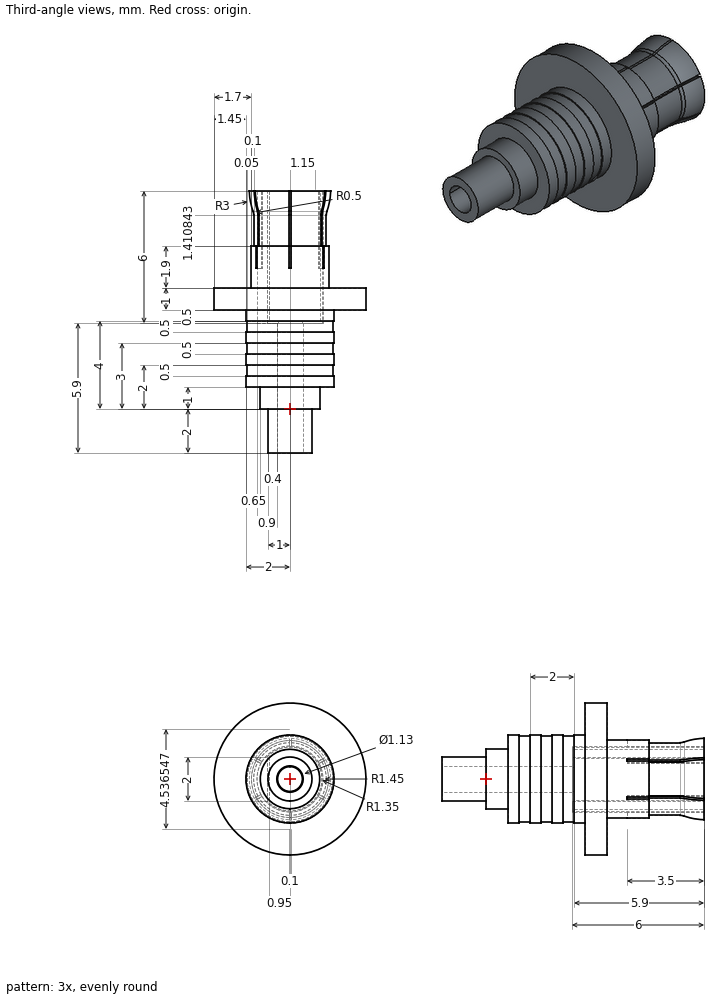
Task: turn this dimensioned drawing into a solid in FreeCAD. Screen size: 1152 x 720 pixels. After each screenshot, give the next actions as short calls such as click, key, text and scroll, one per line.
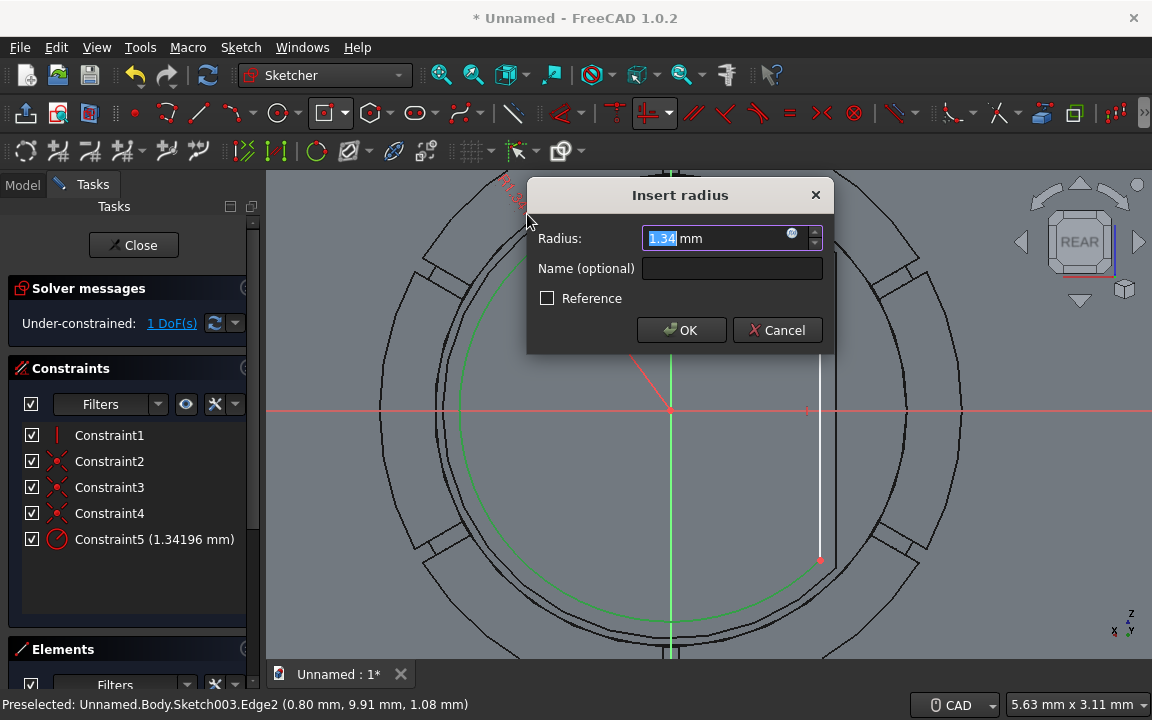
text(1.35)
key(Return)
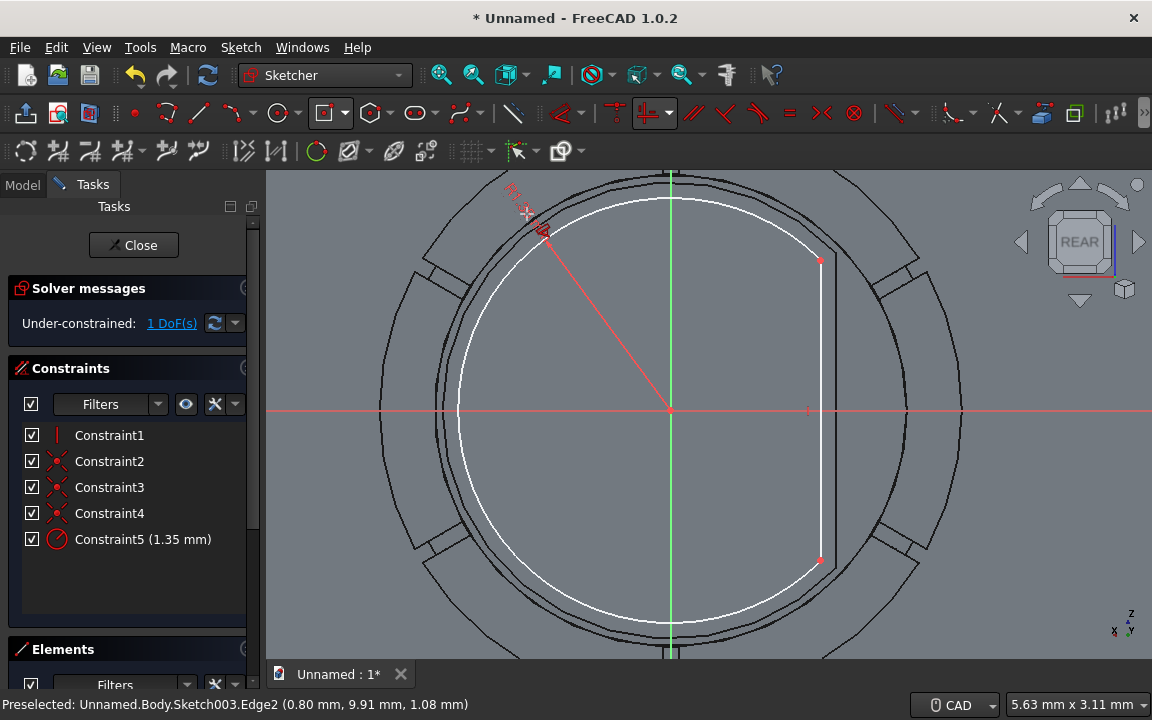
click(821, 561)
click(746, 595)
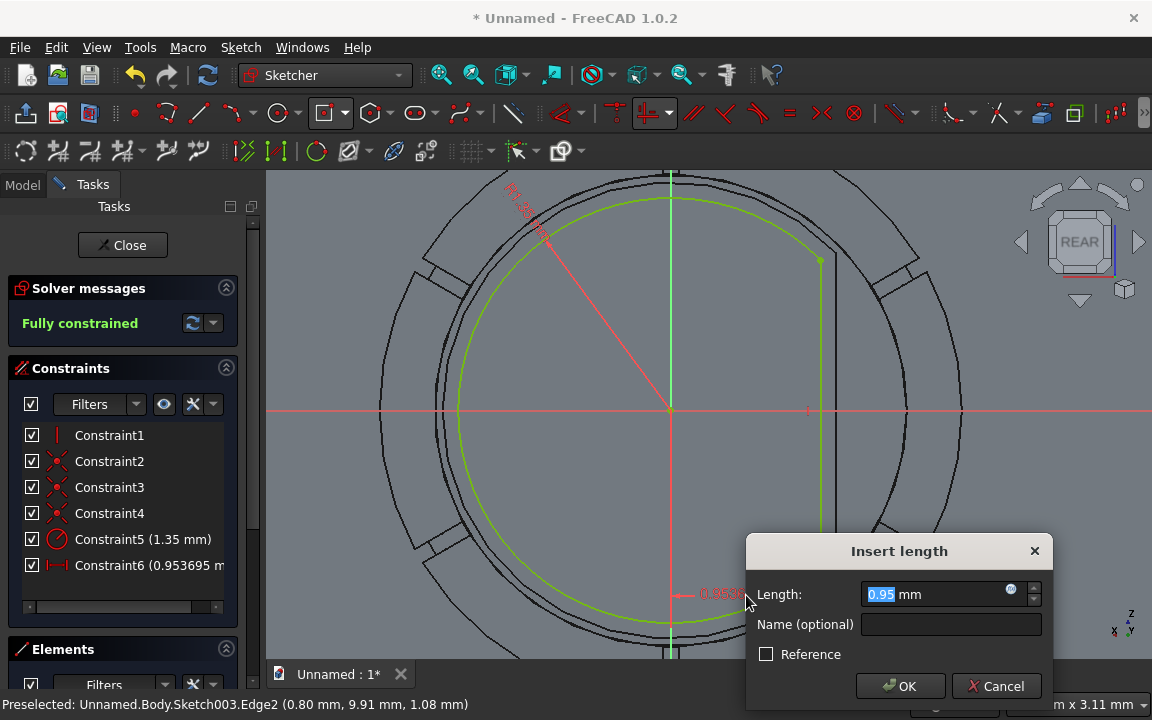
text(0.95)
key(Return)
key(Escape)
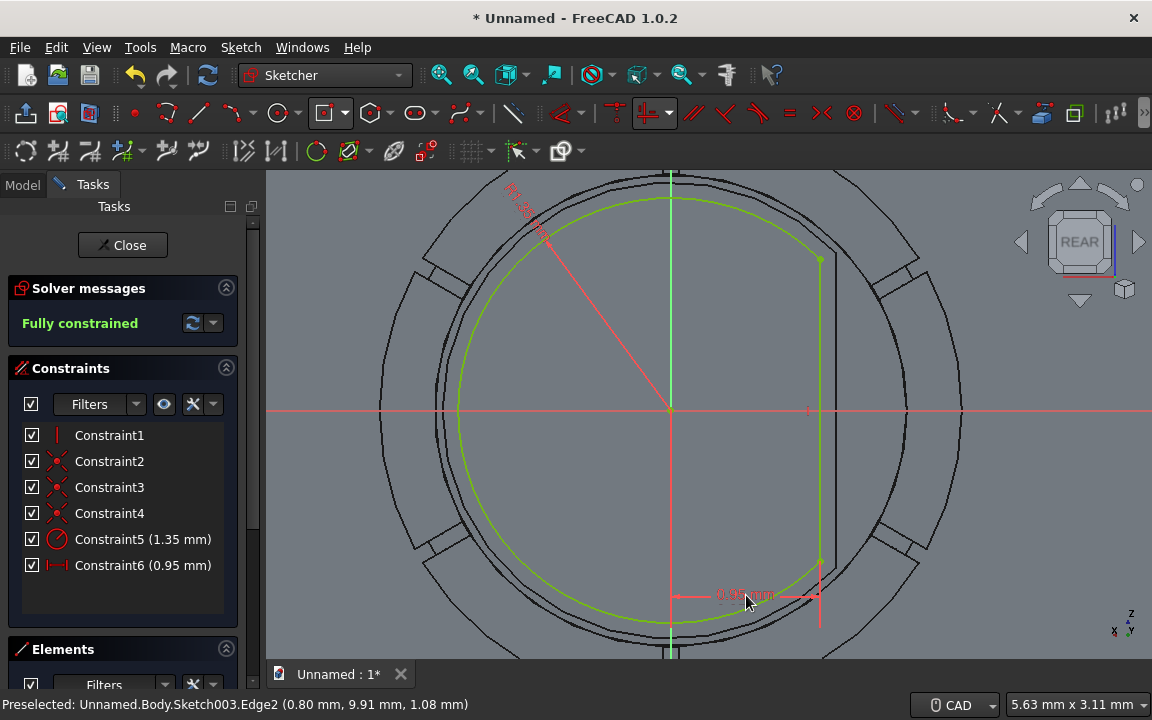
click(123, 245)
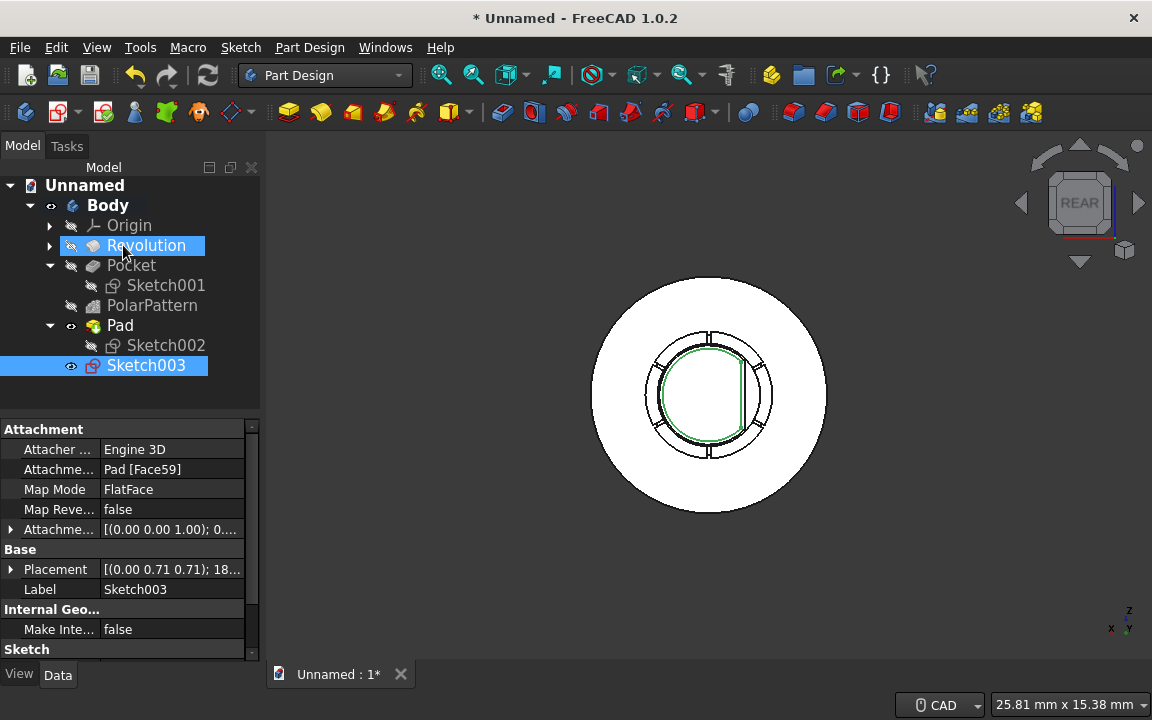
click(504, 112)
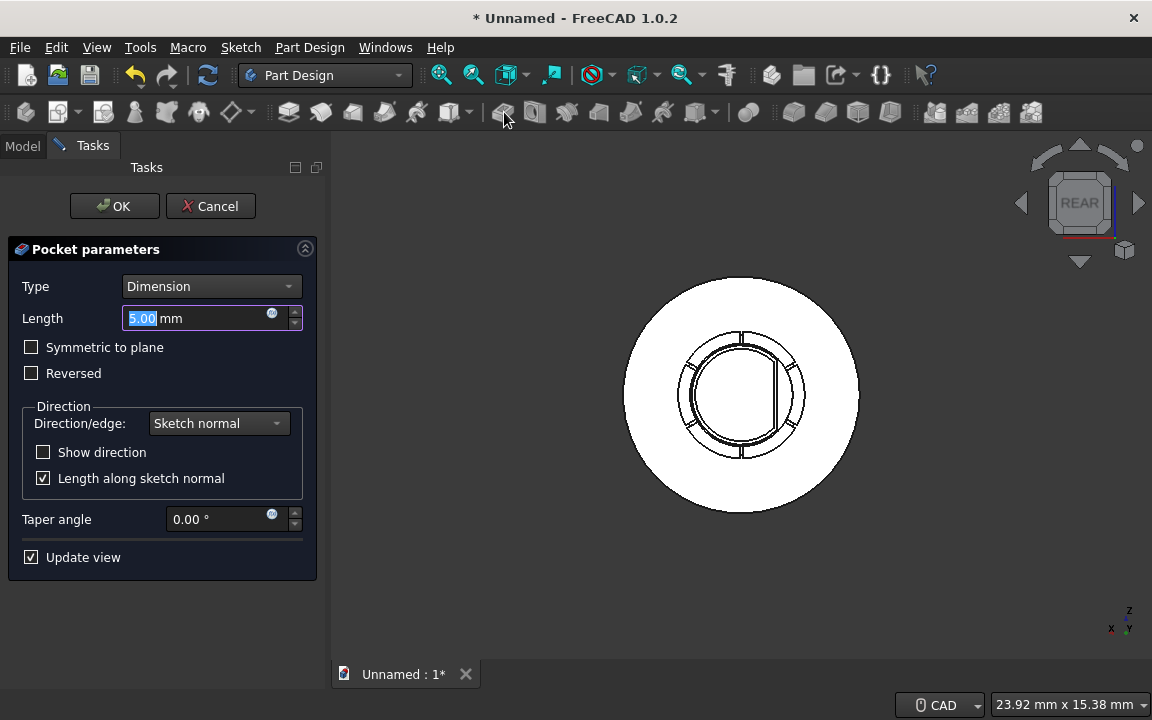
text(5.9)
key(Tab)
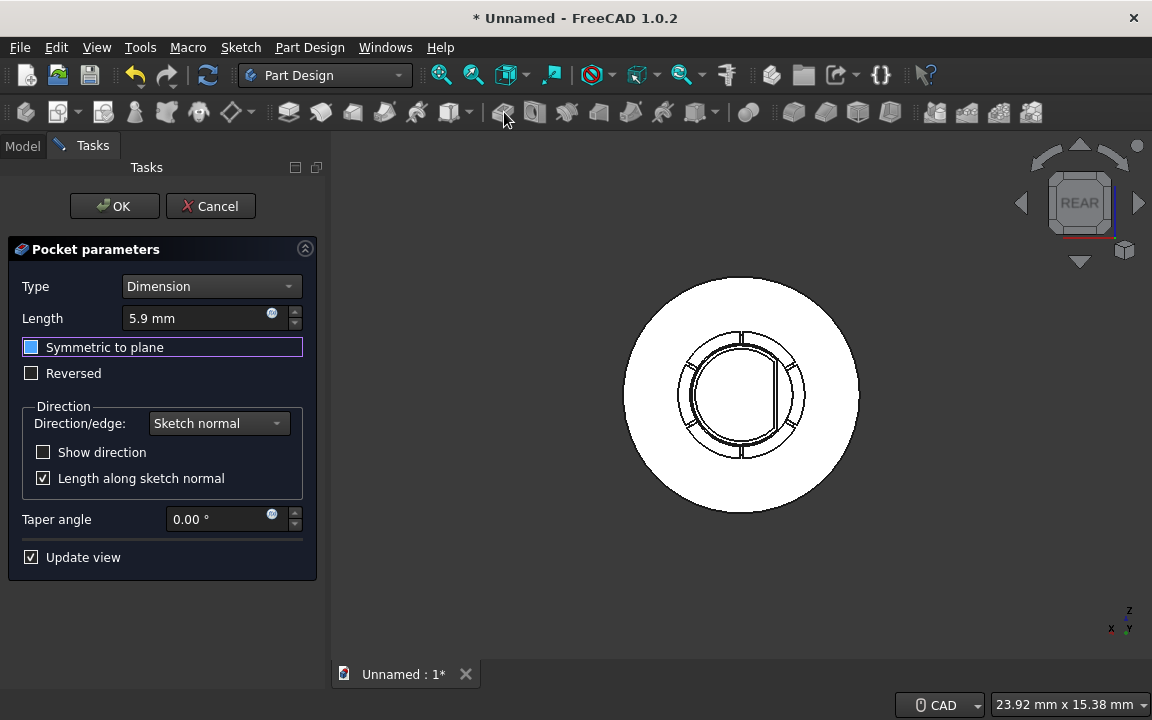
click(115, 206)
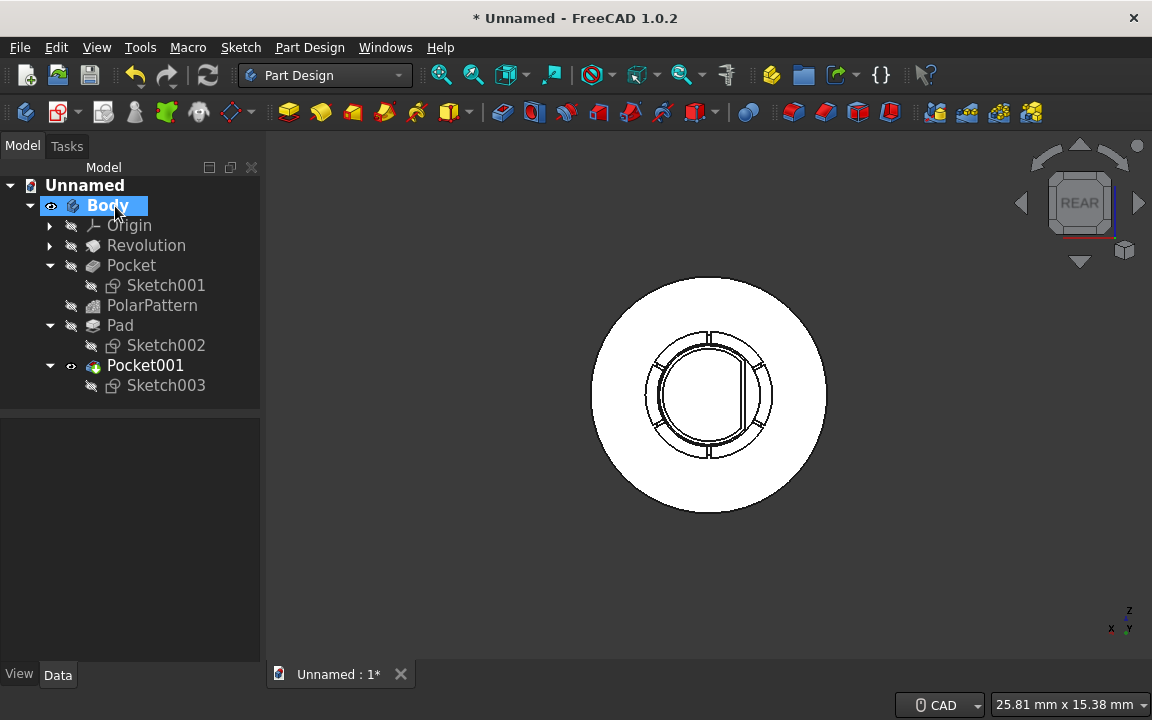
click(442, 76)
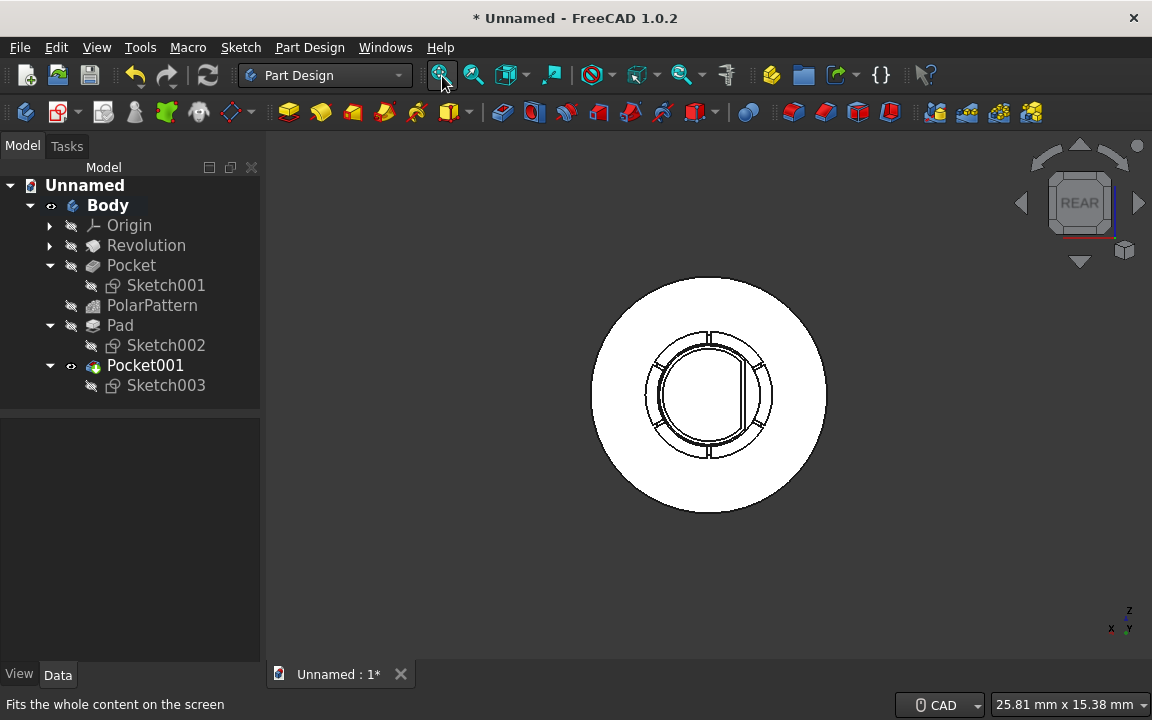
click(702, 394)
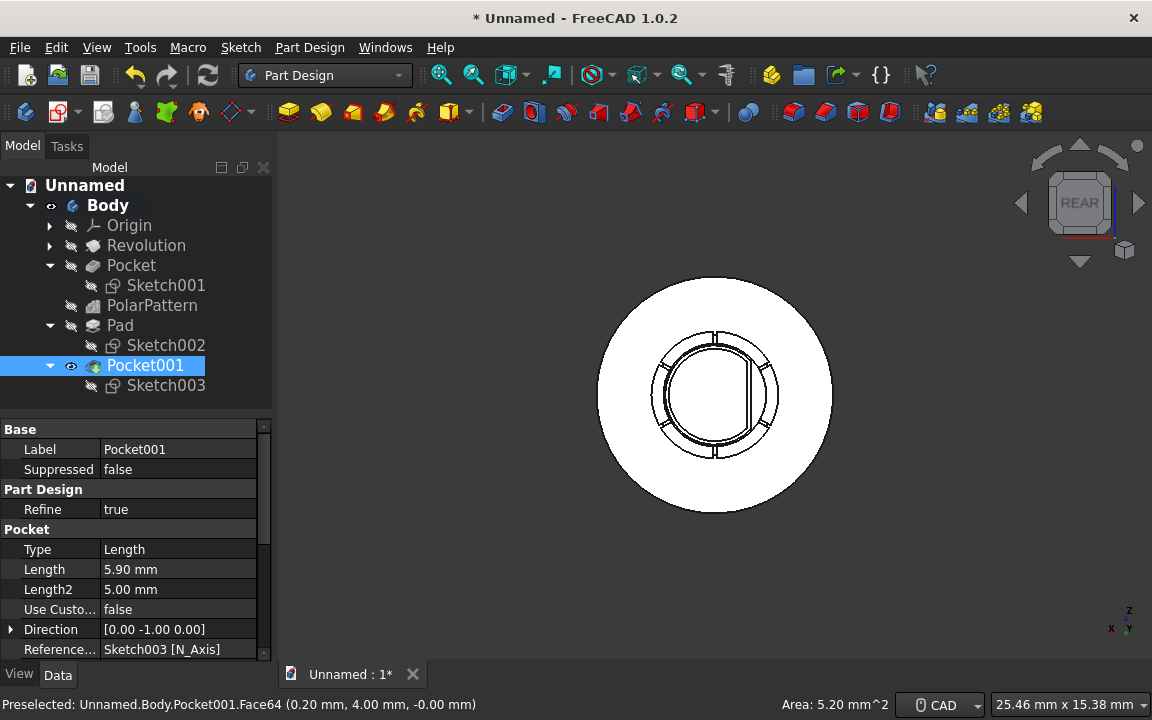
click(58, 112)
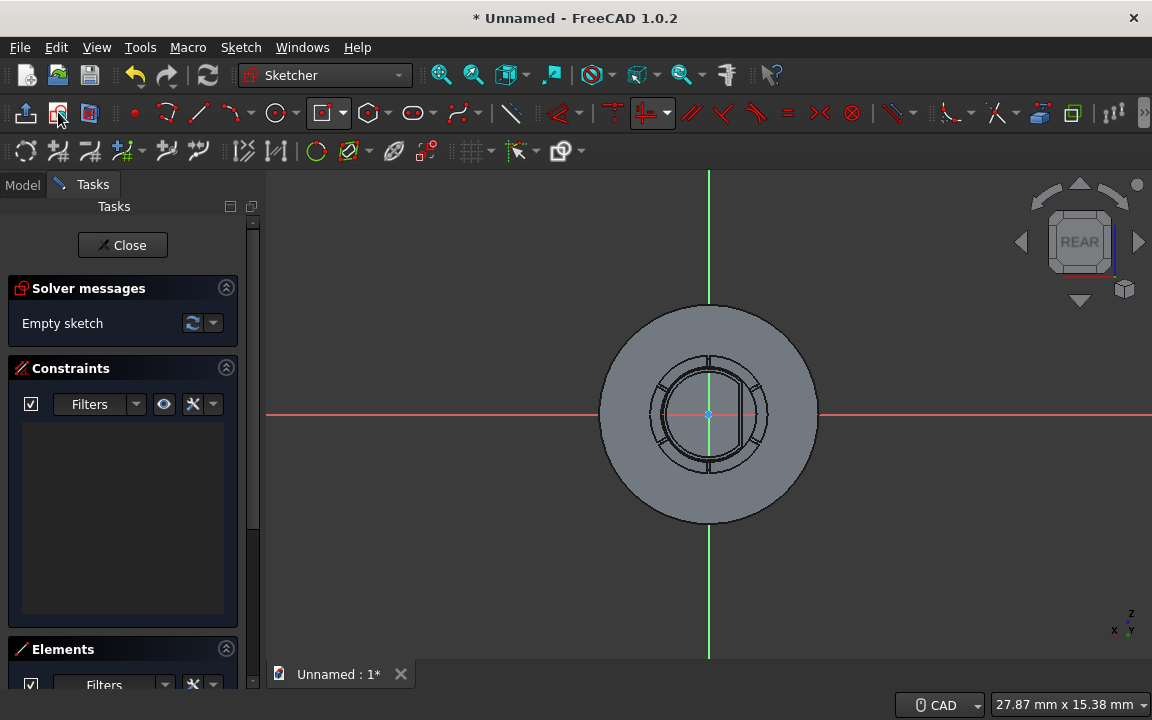
click(90, 114)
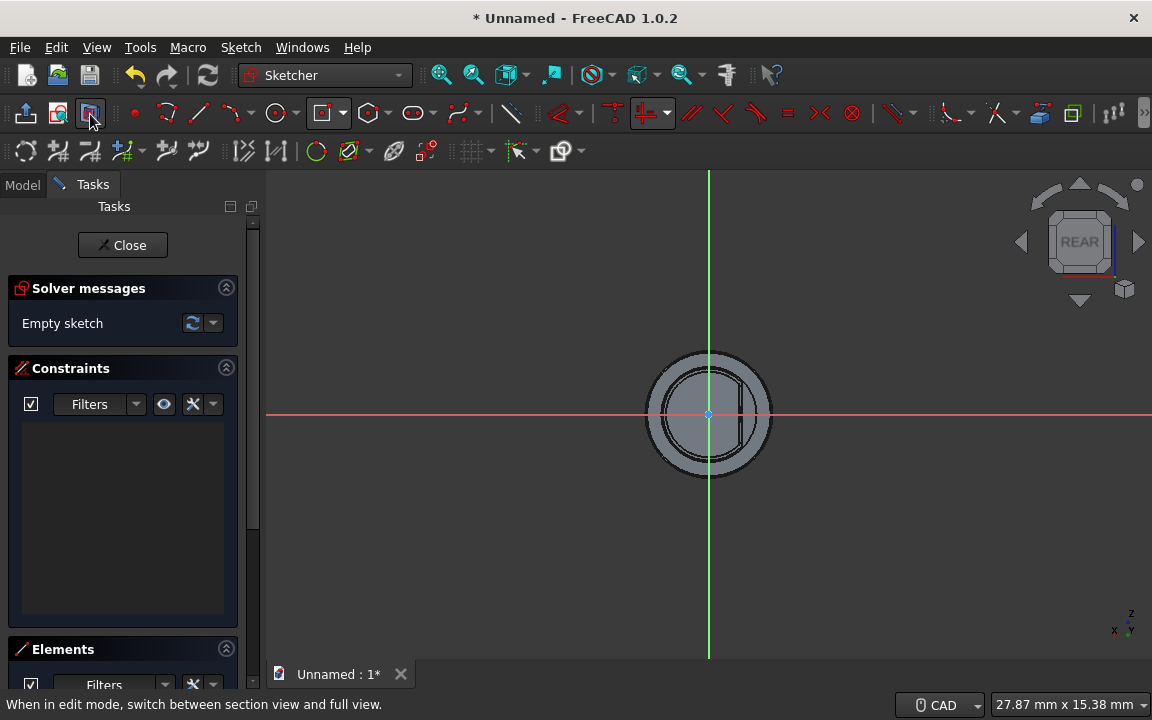
scroll(717, 414, up, 11)